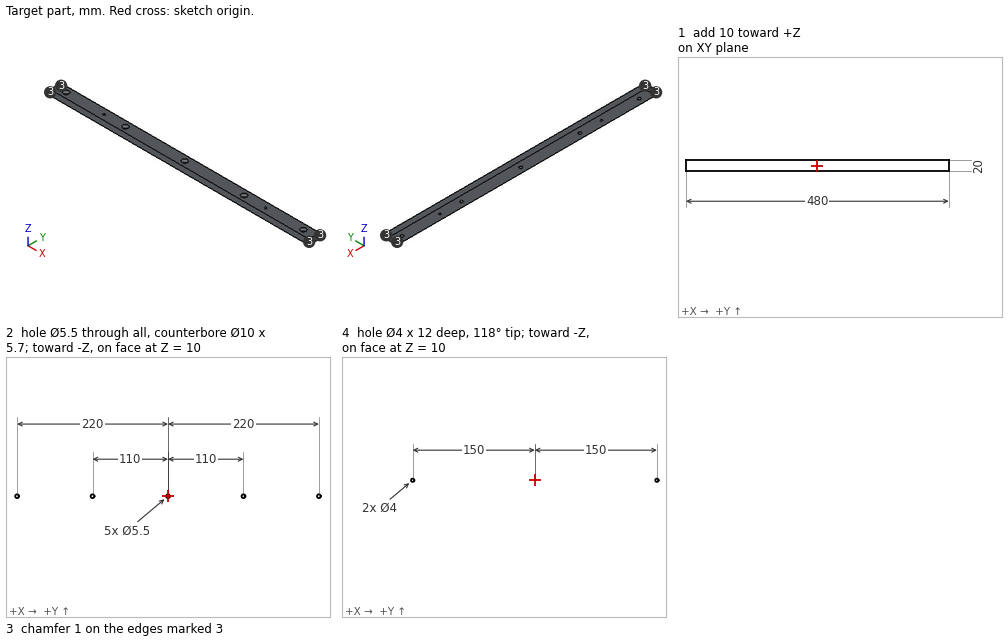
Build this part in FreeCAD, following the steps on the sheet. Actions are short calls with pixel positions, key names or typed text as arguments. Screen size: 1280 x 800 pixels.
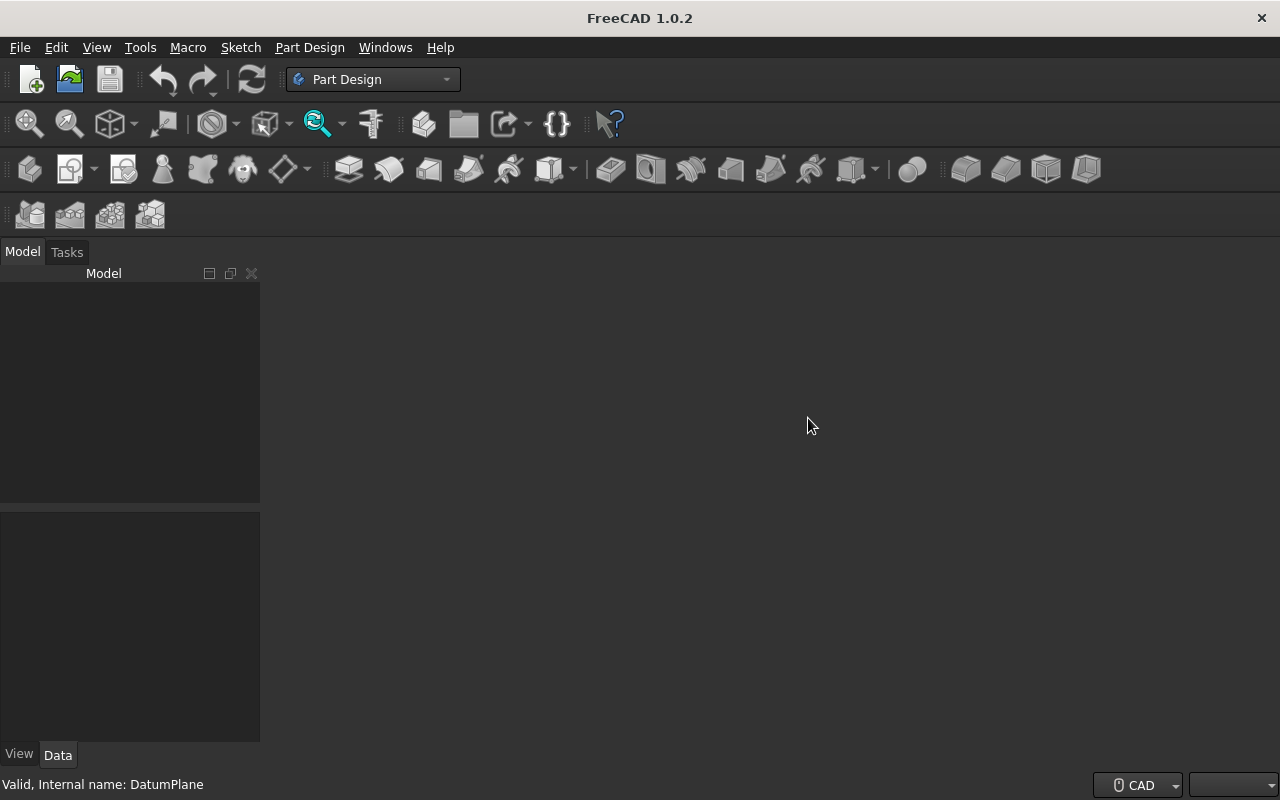
click(30, 80)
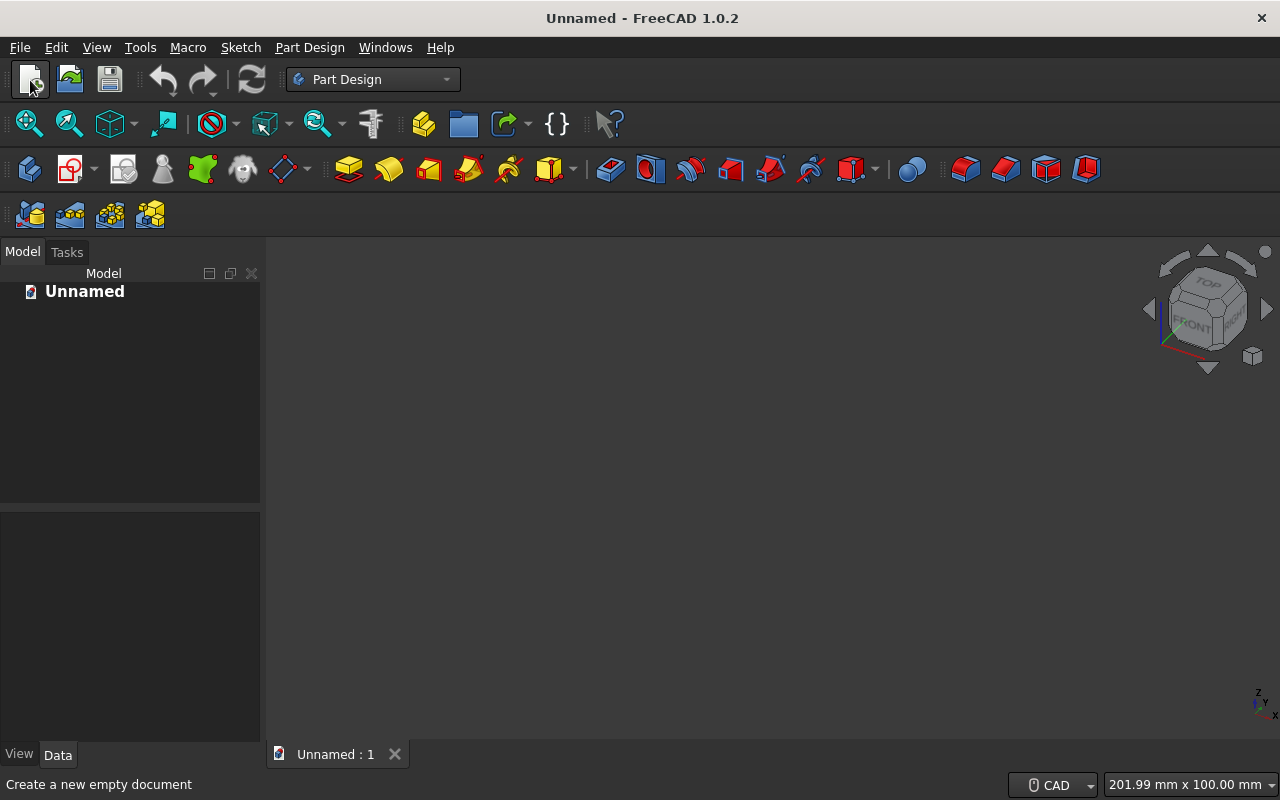
click(70, 170)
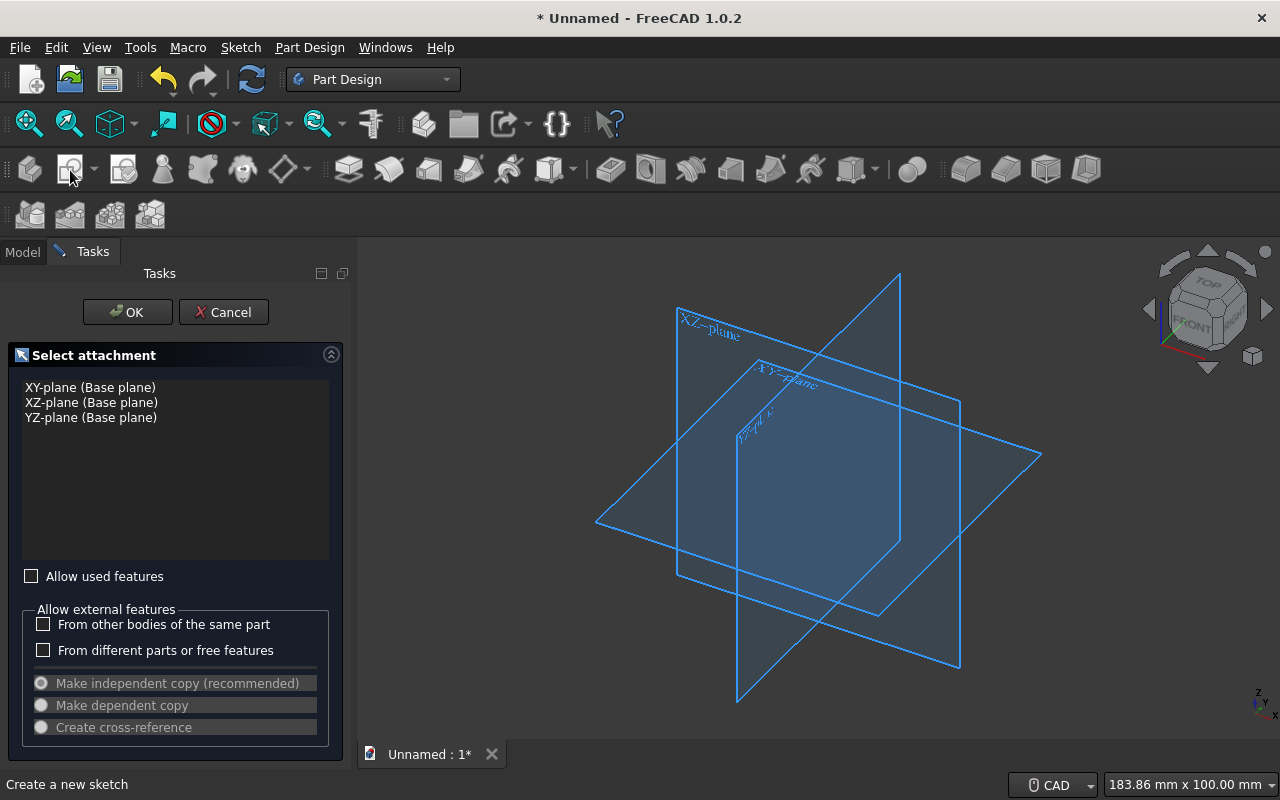
click(82, 388)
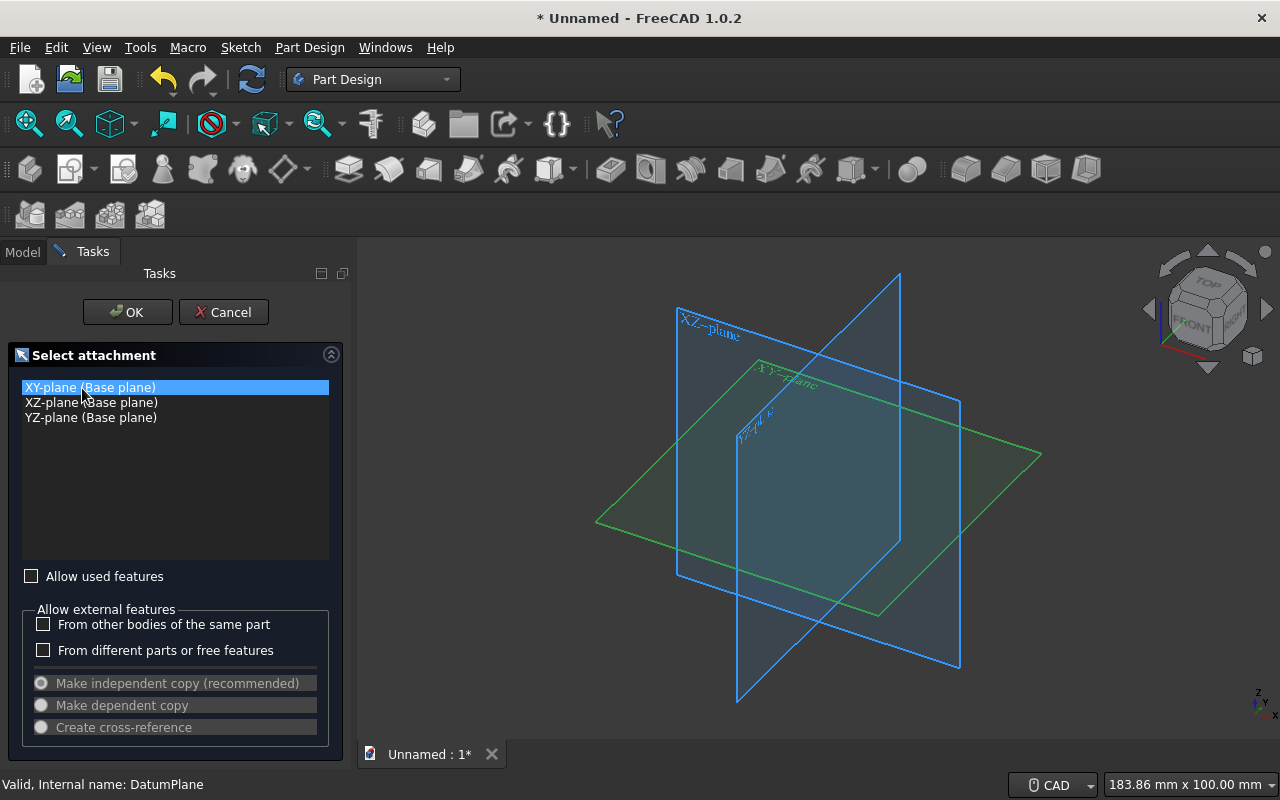
click(128, 312)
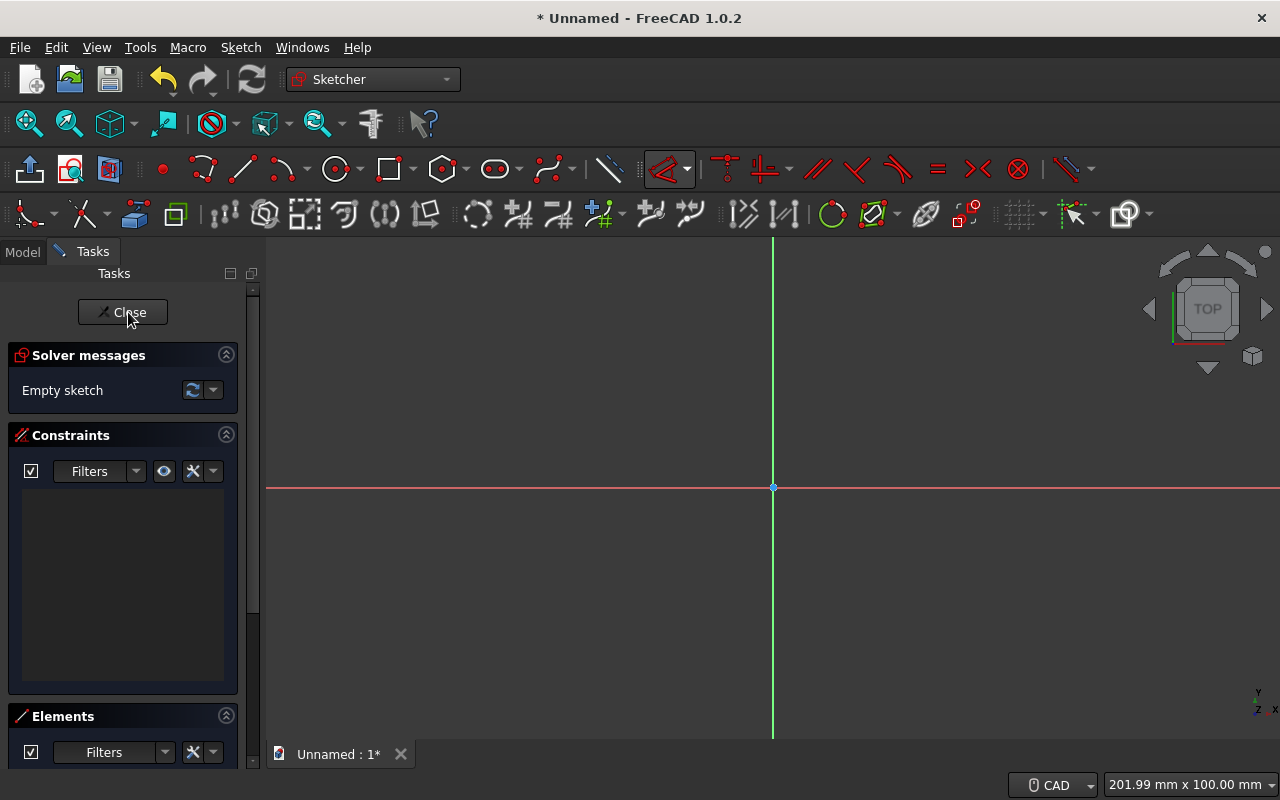
scroll(682, 488, down, 7)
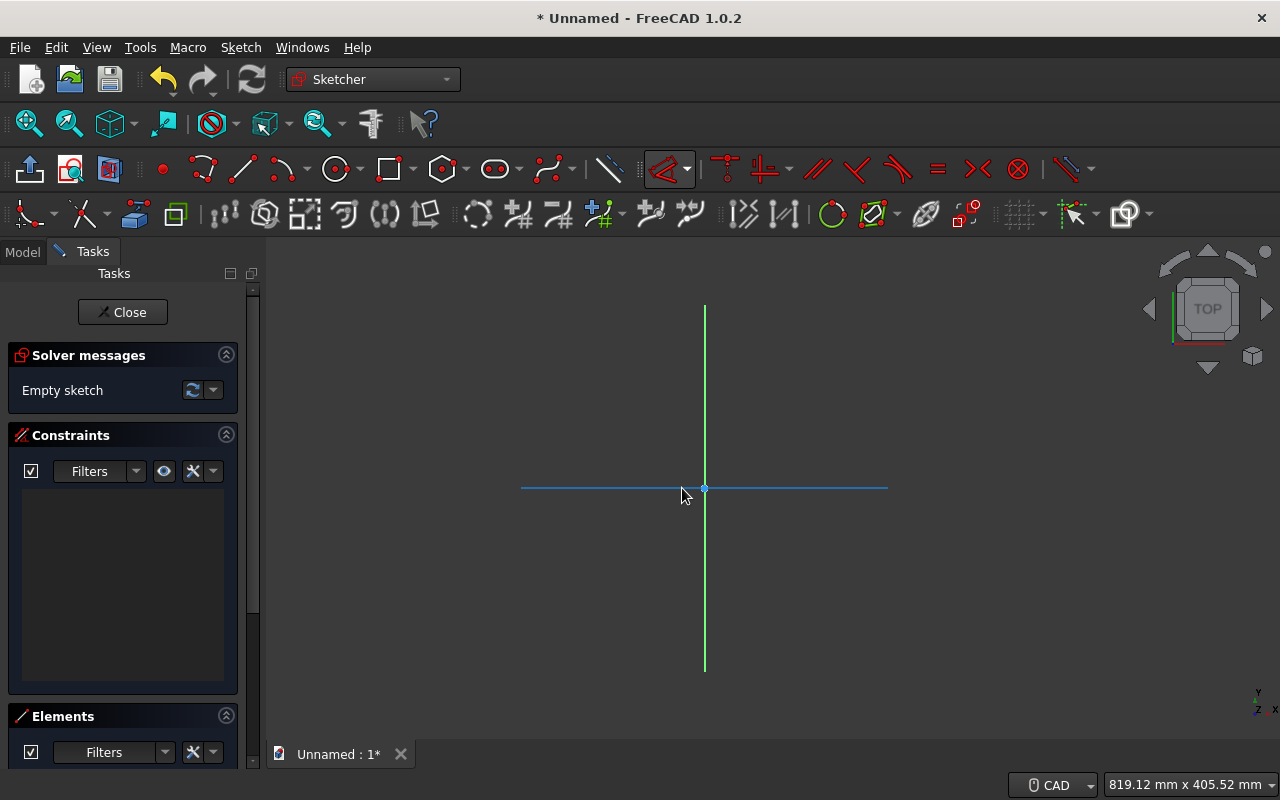
click(416, 170)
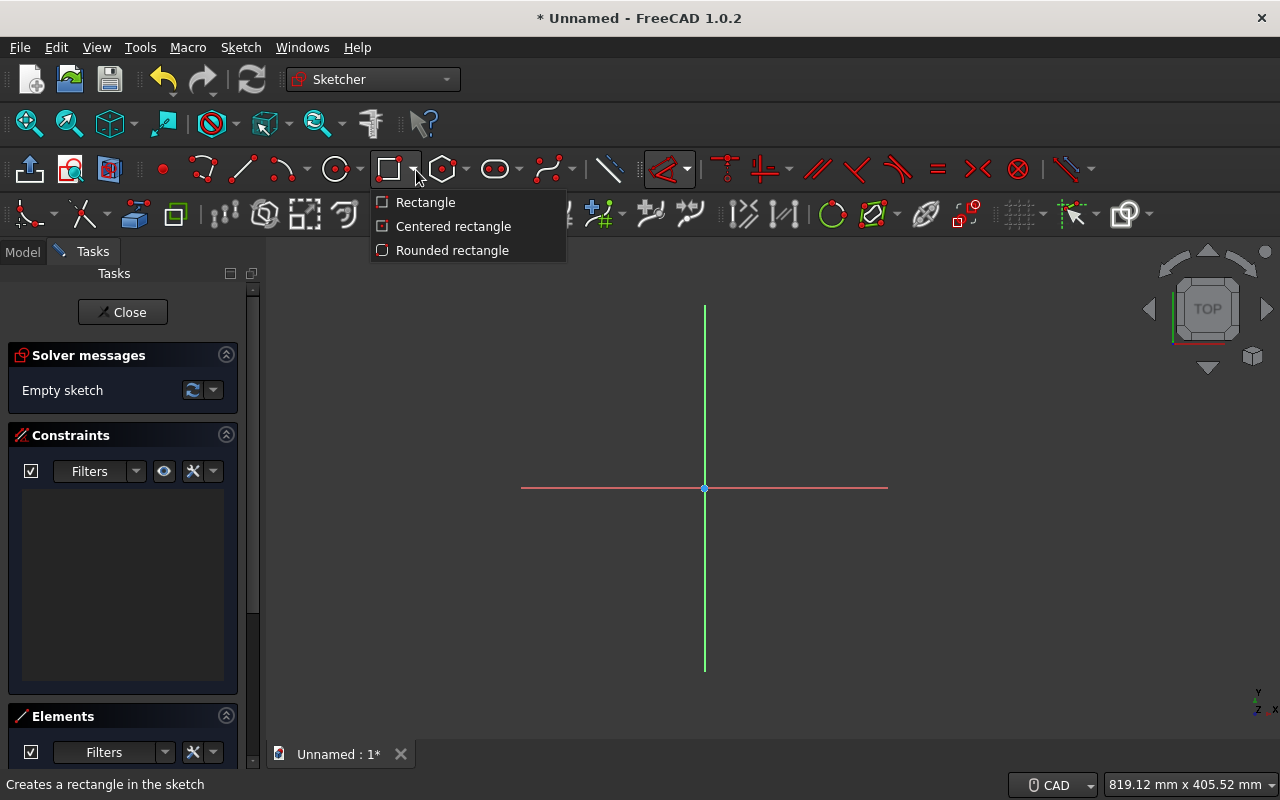
click(468, 226)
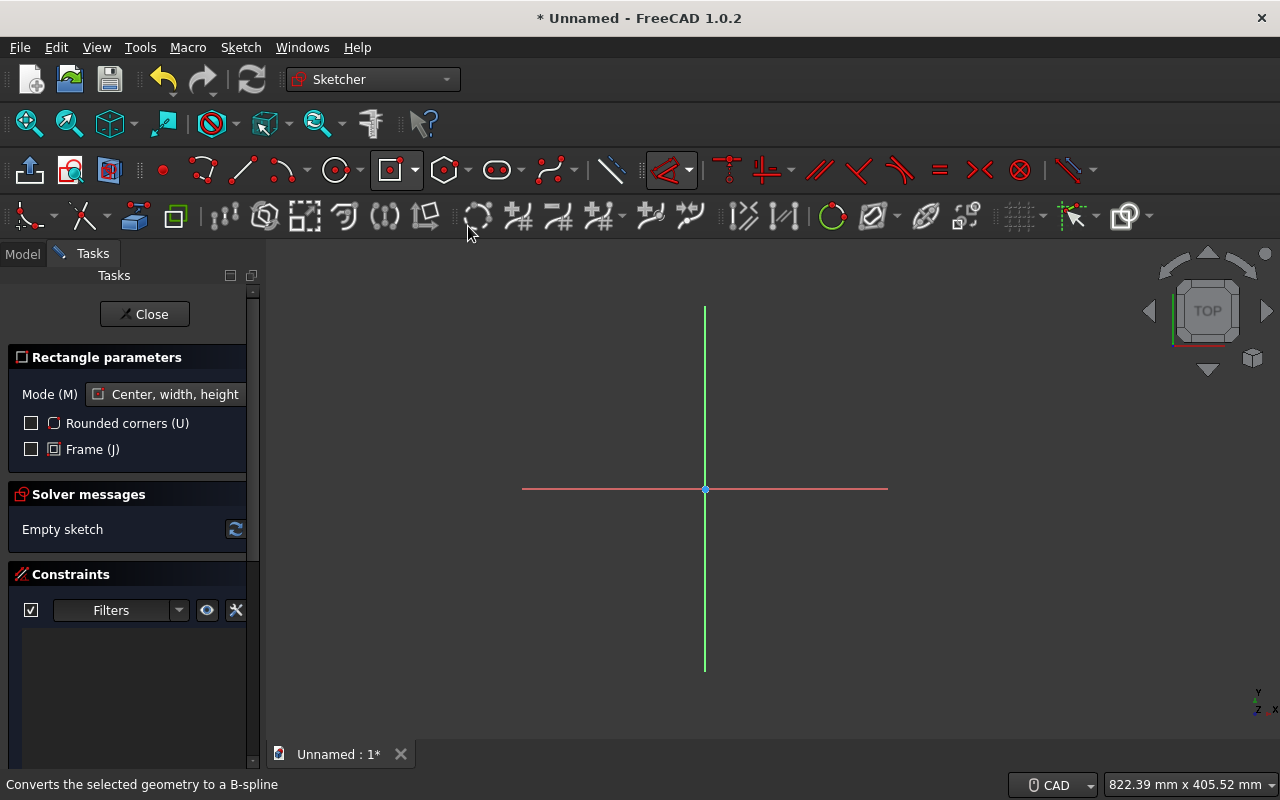
scroll(705, 489, up, 2)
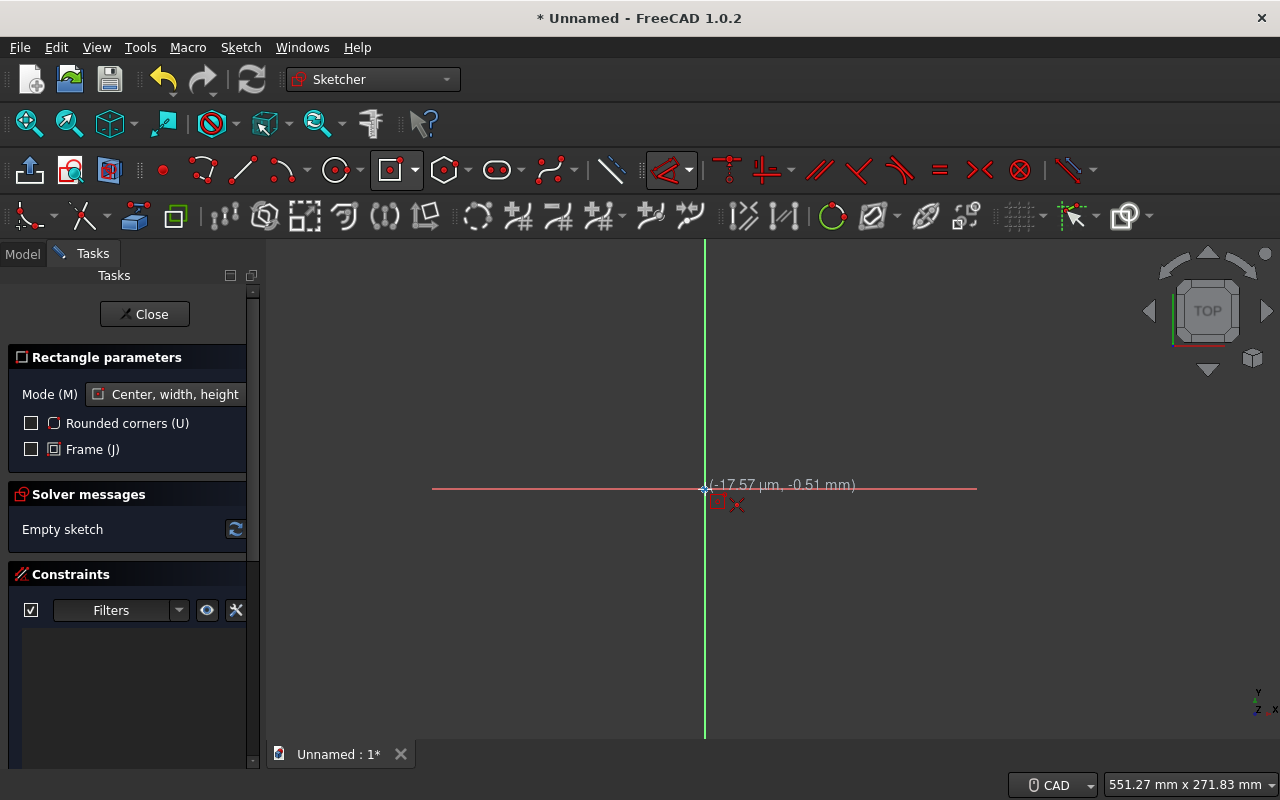
click(705, 489)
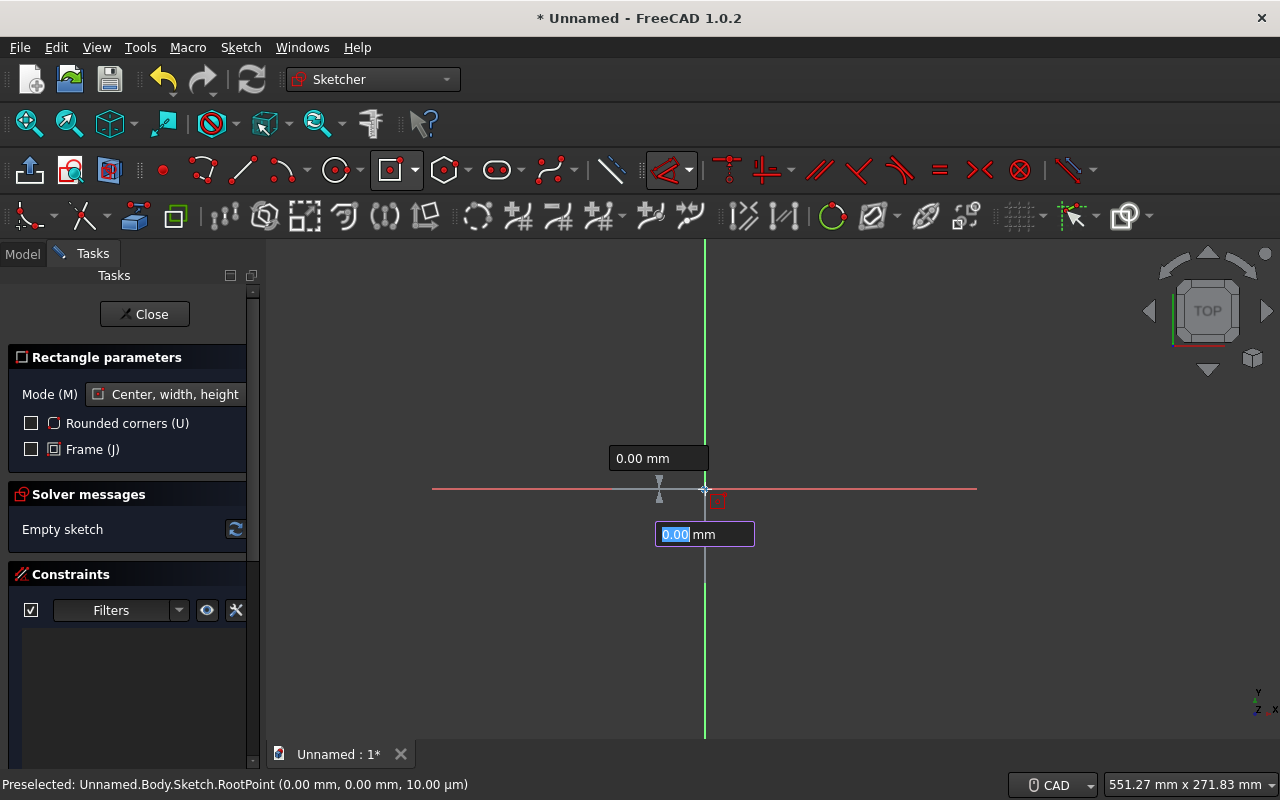
scroll(704, 488, down, 2)